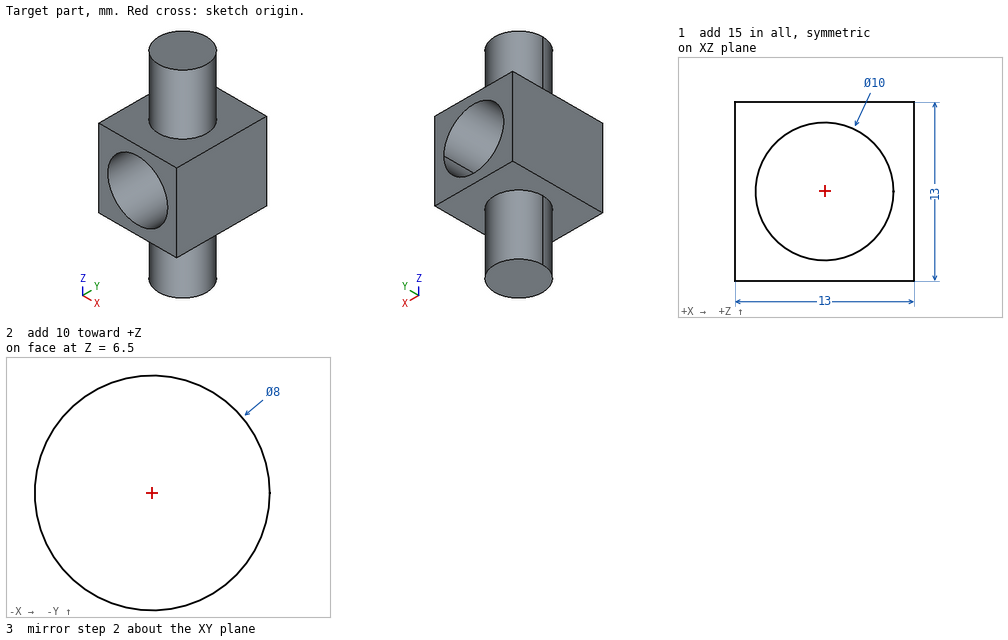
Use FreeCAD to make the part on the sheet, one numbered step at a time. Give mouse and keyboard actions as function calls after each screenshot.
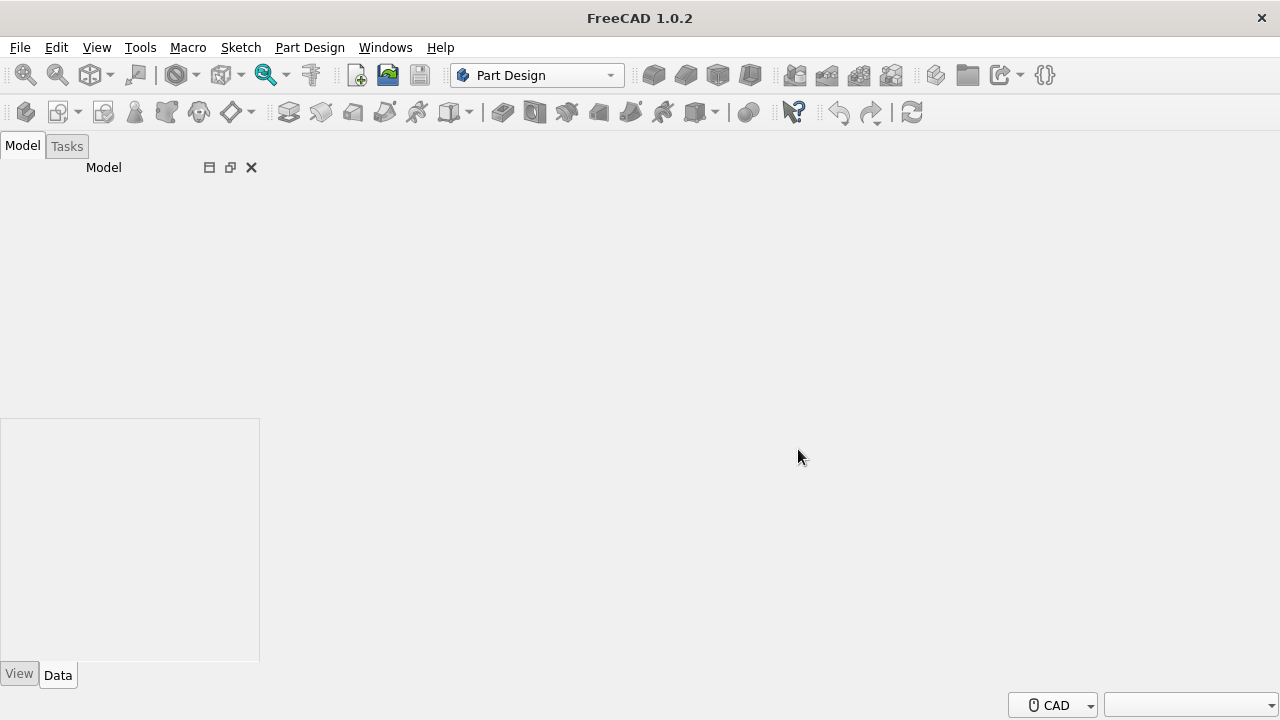
click(356, 76)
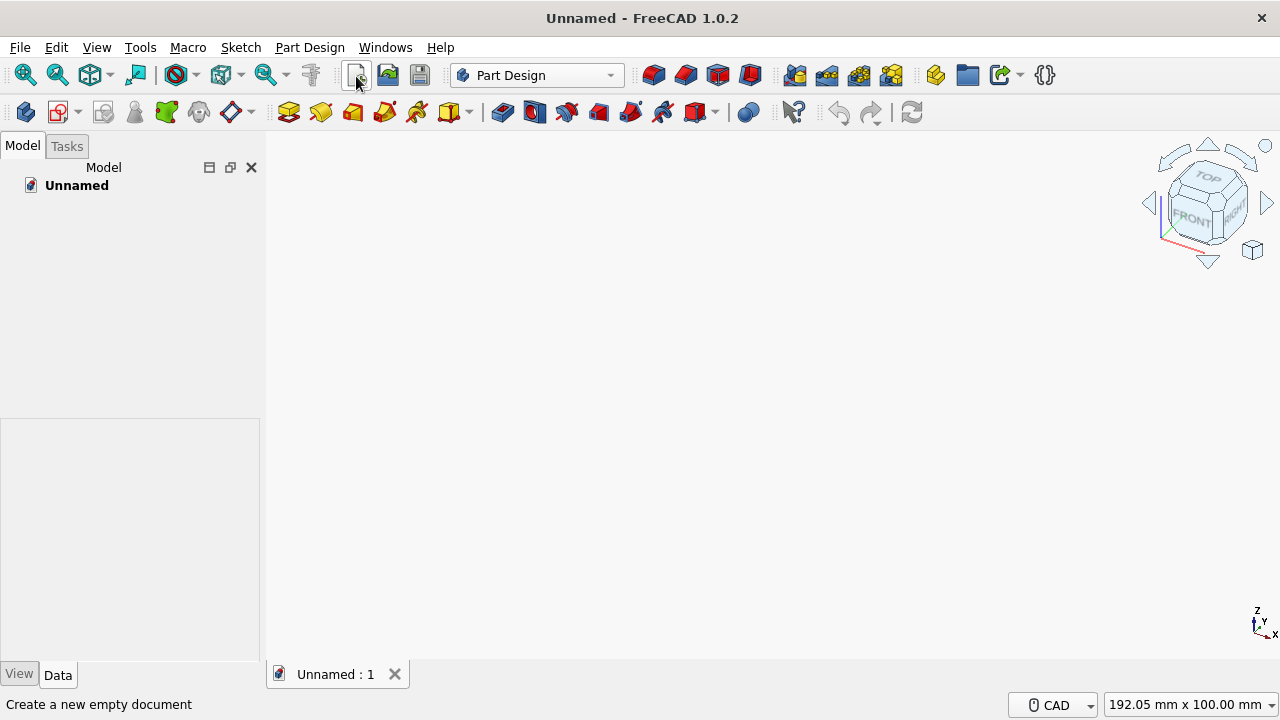
click(58, 112)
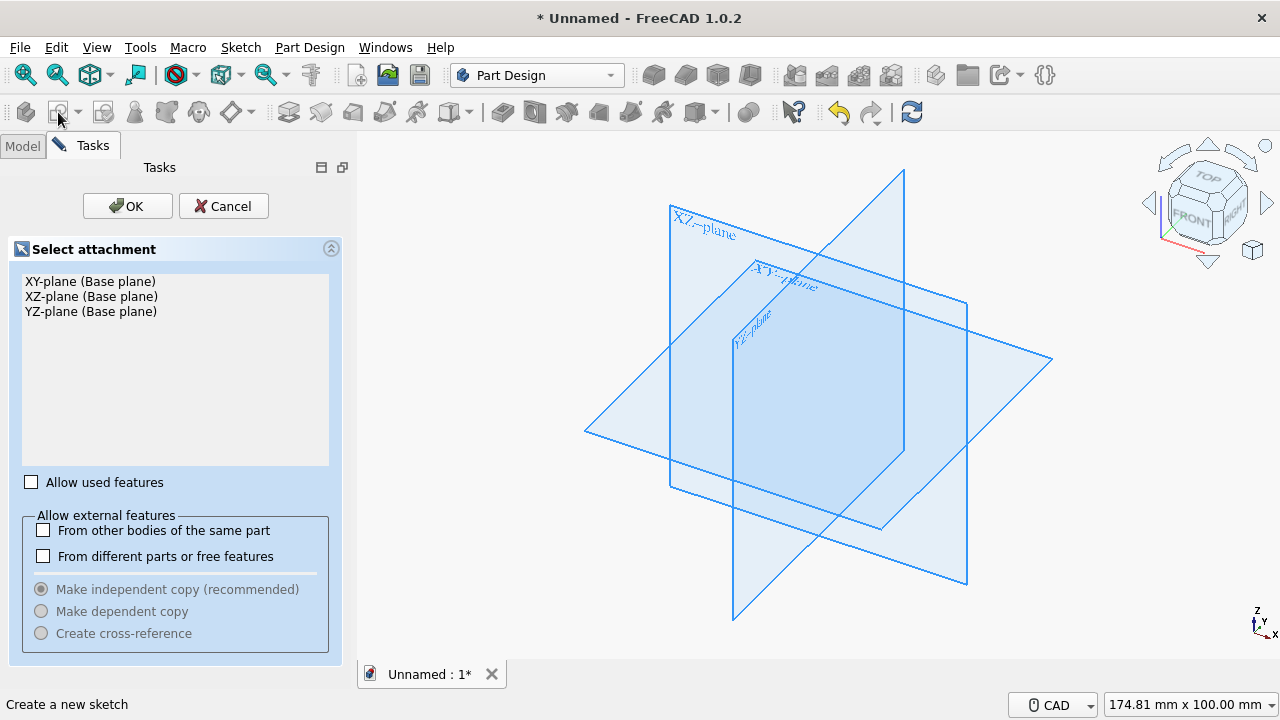
click(82, 296)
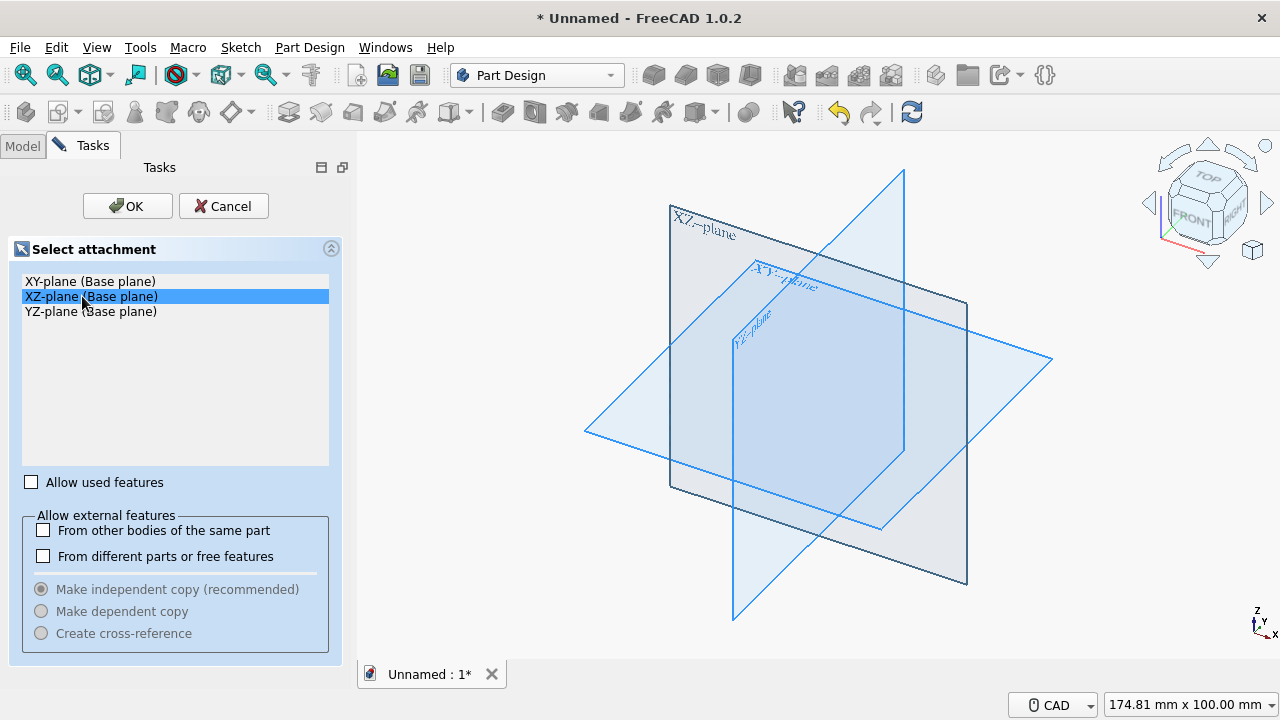
click(128, 206)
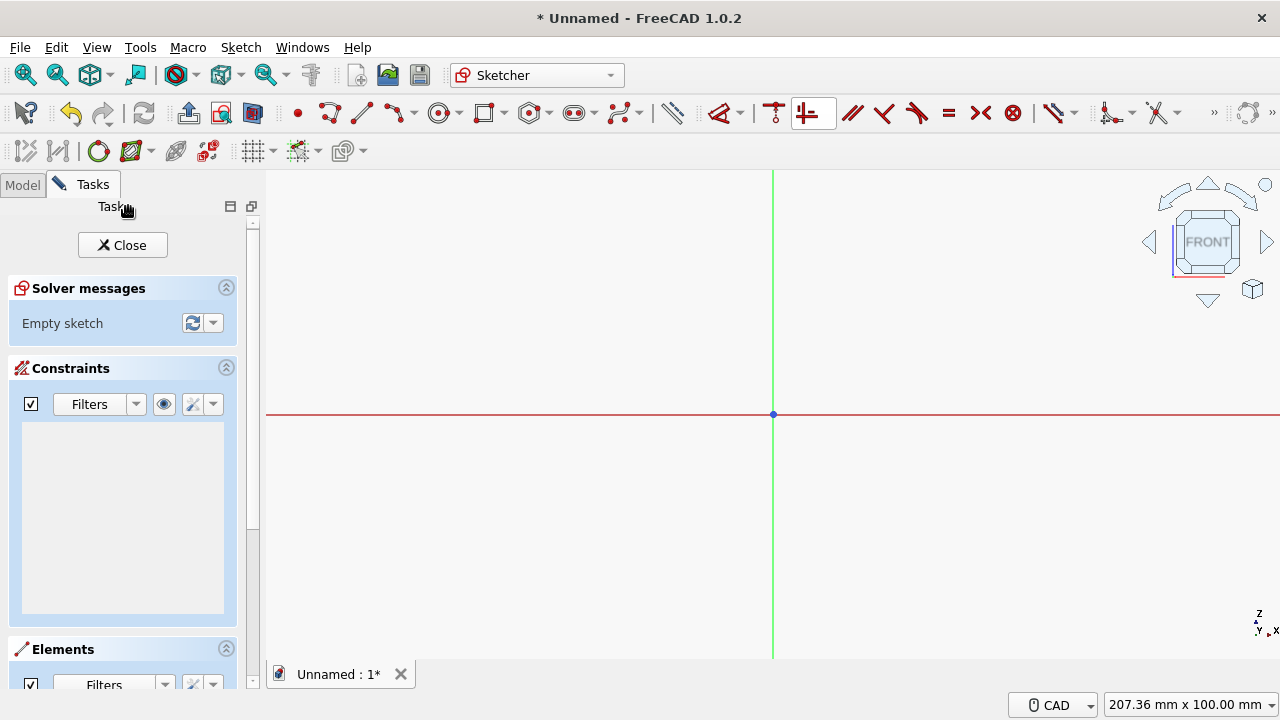
scroll(790, 414, up, 8)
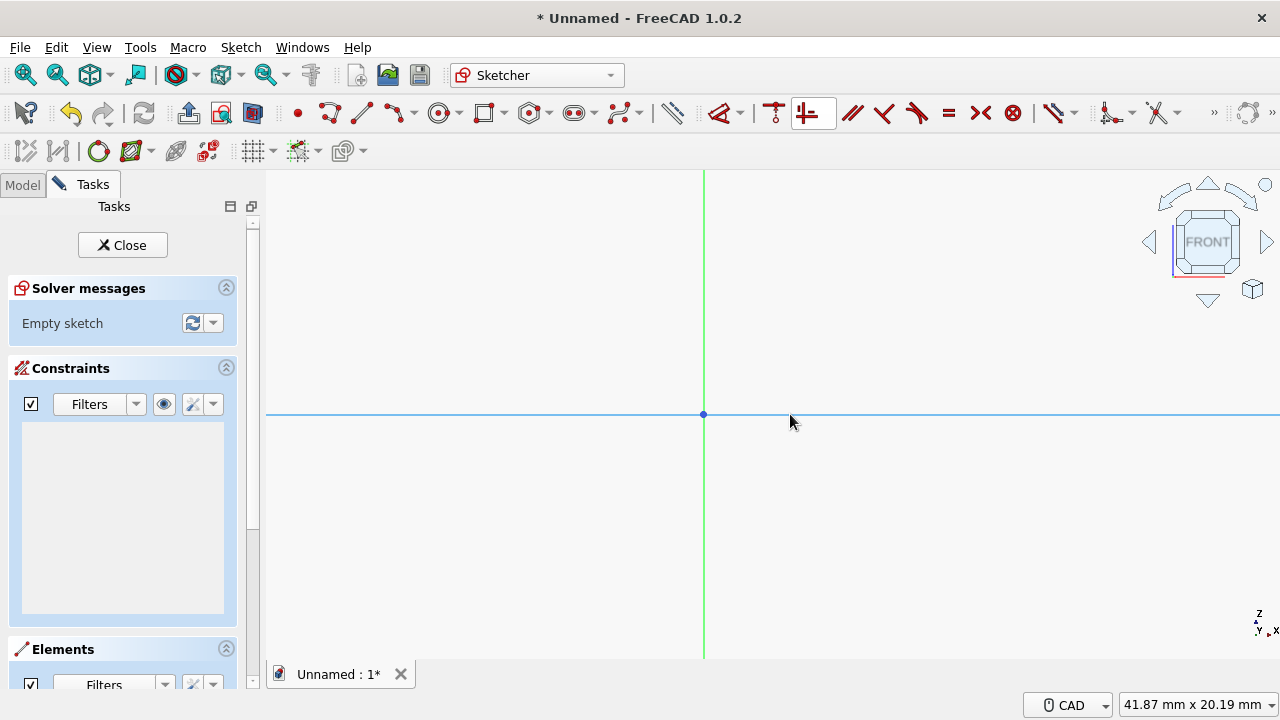
click(506, 114)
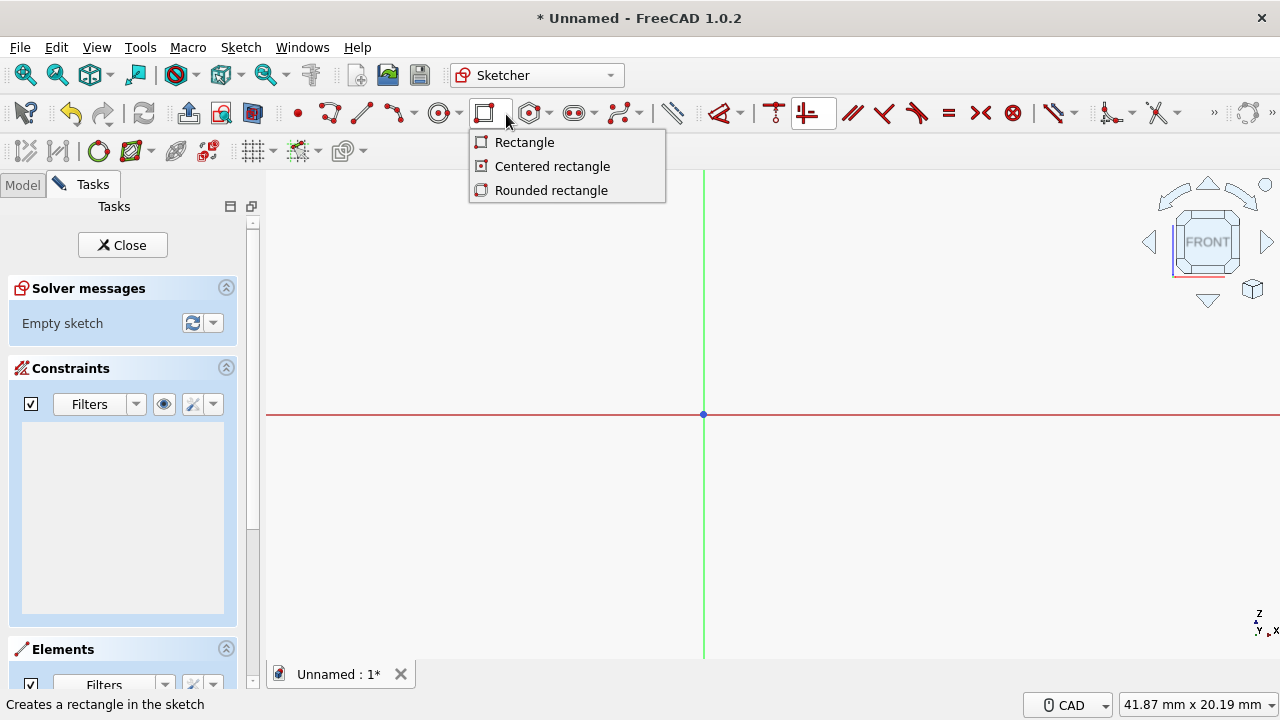
click(568, 166)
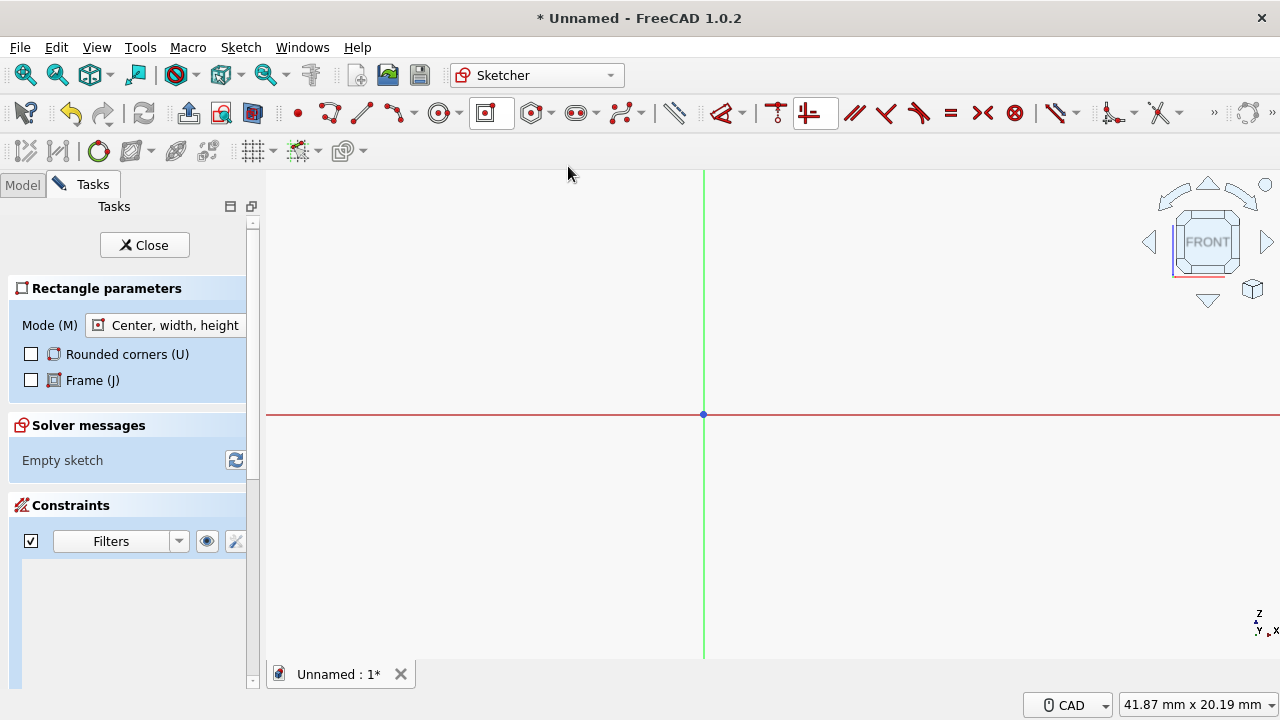
click(704, 414)
move(861, 257)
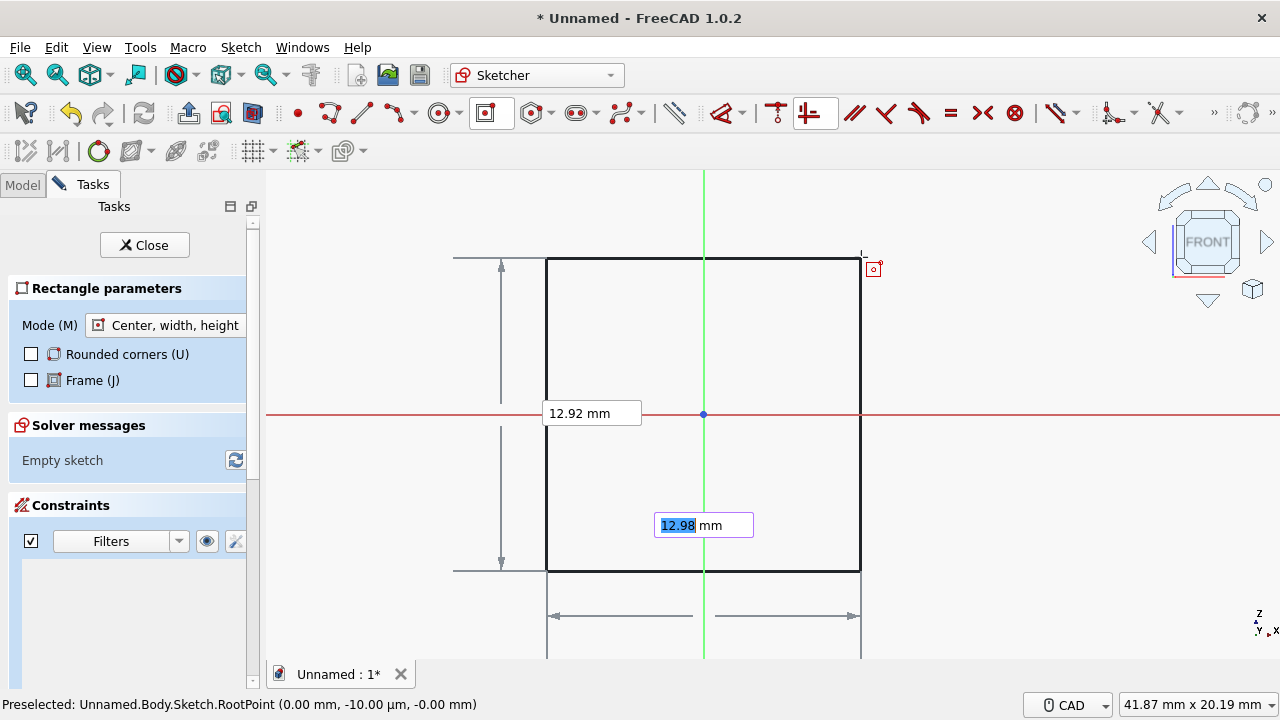
text(13)
key(Tab)
text(13)
key(Return)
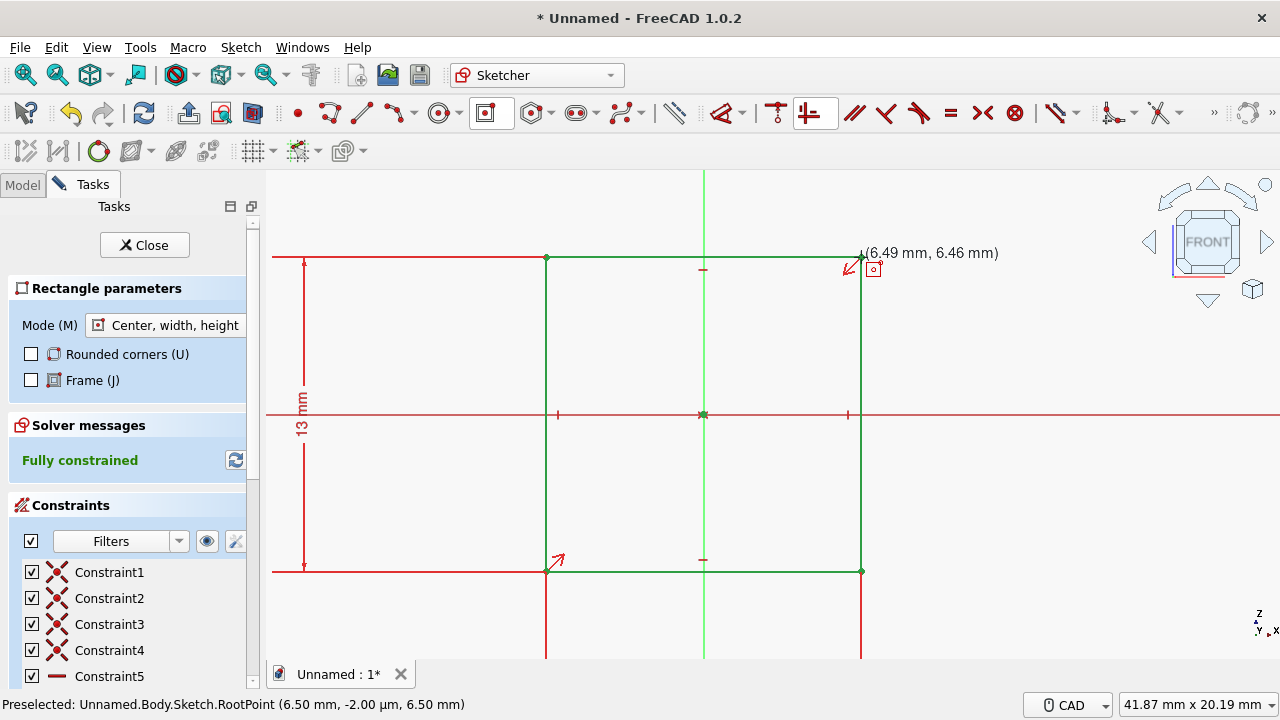
click(440, 114)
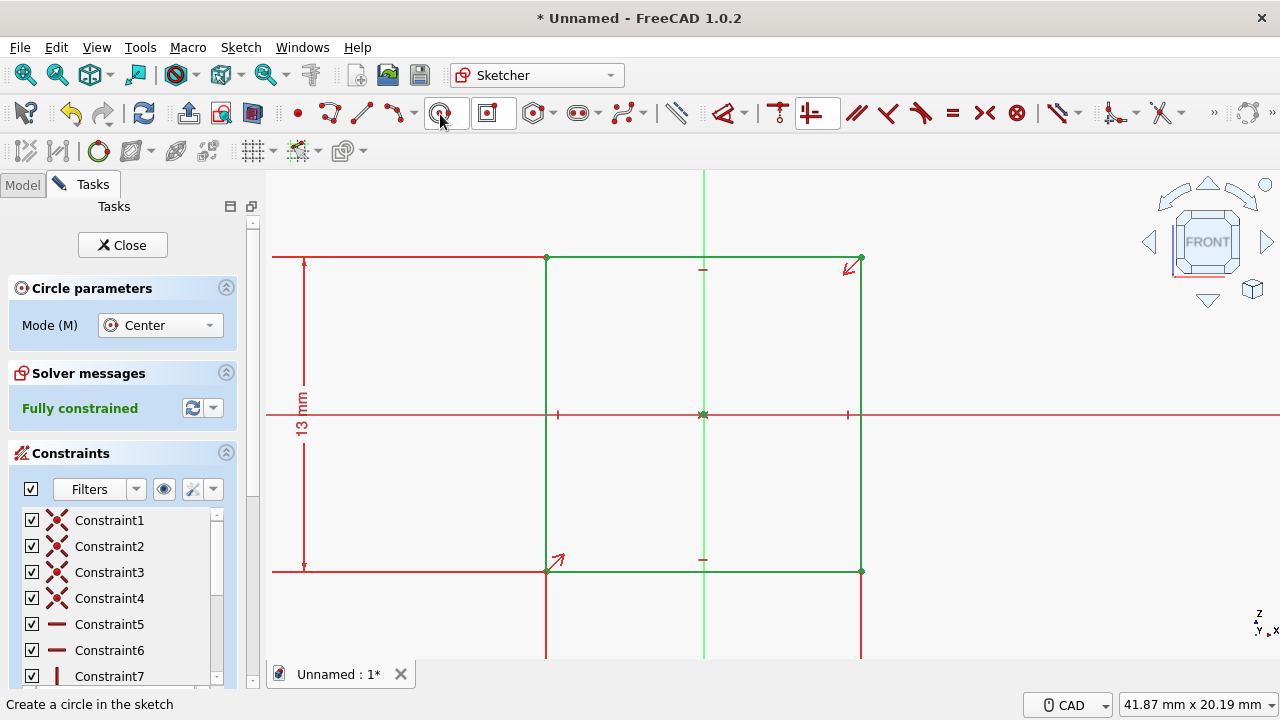
click(704, 414)
move(789, 329)